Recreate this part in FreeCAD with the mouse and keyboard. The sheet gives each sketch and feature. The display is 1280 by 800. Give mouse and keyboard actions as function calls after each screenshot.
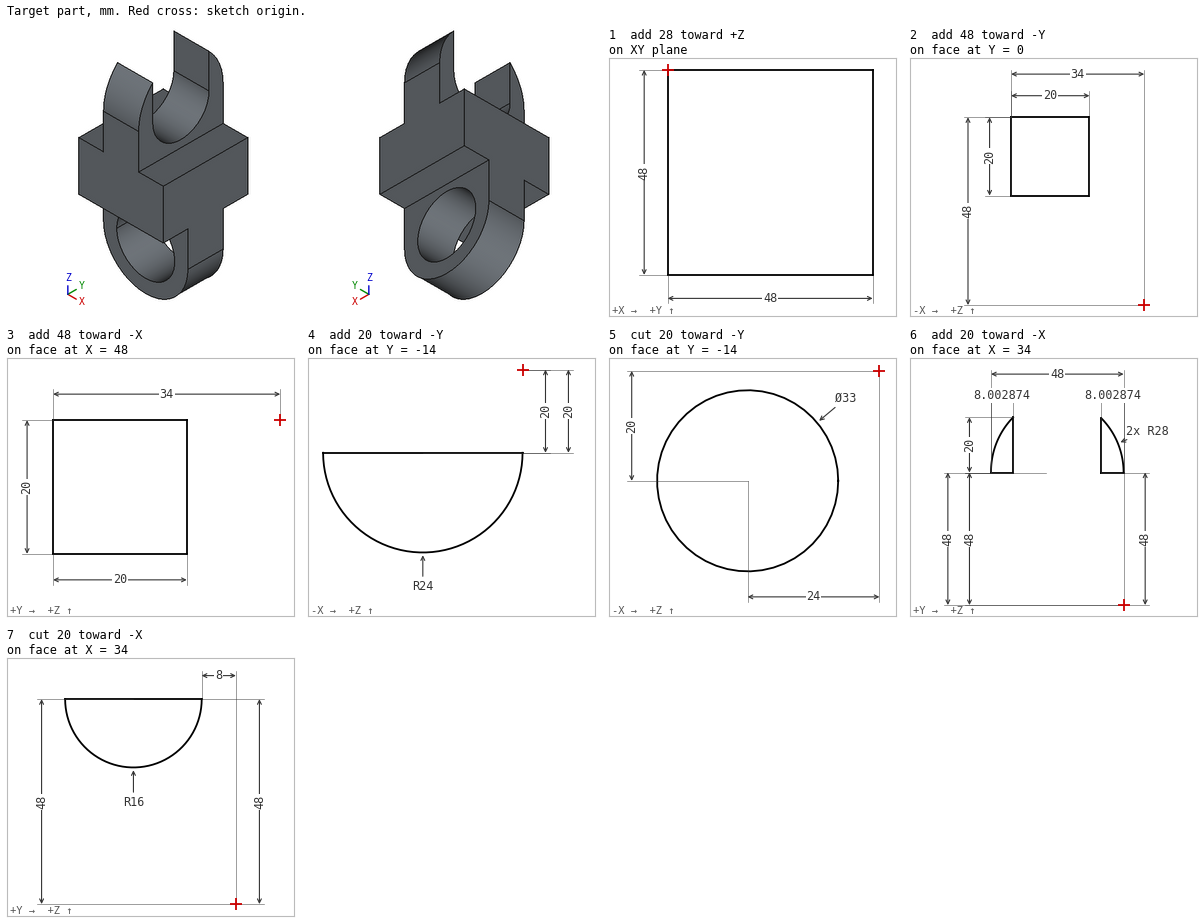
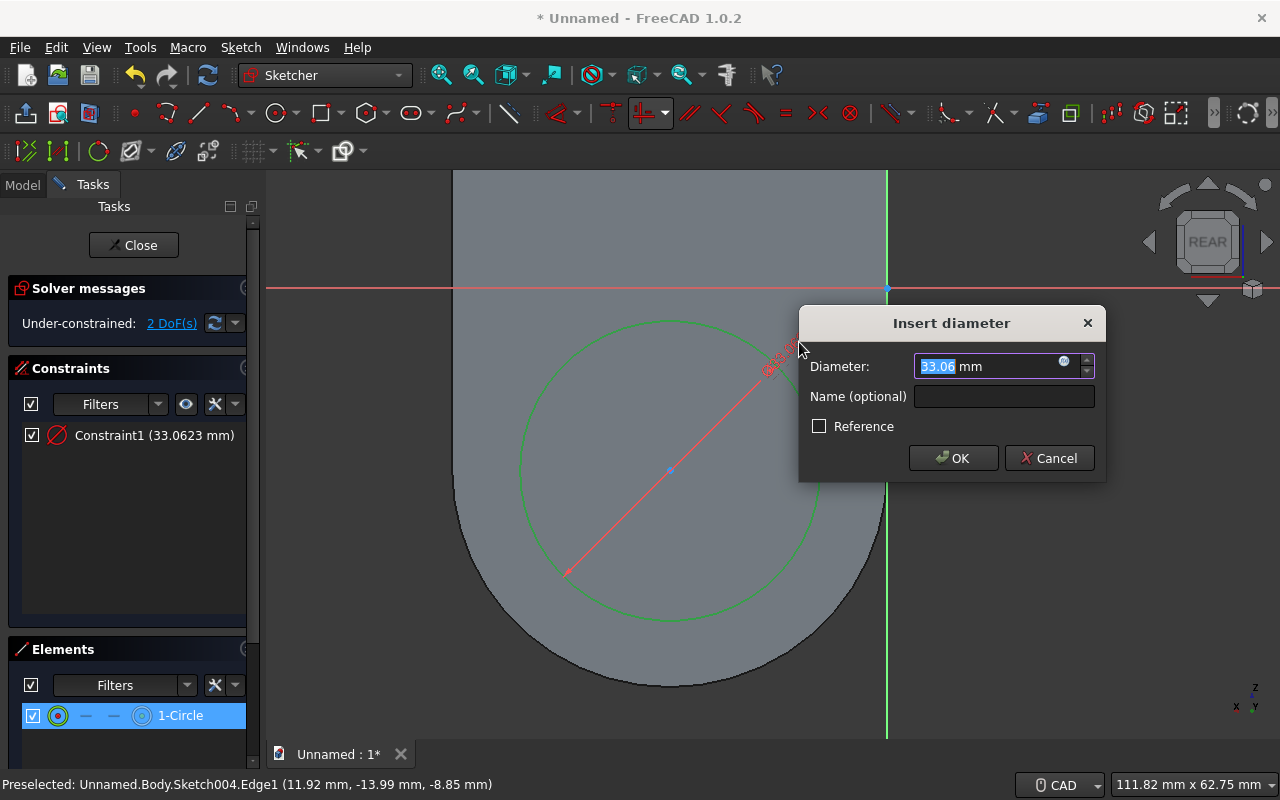
text(33)
key(Return)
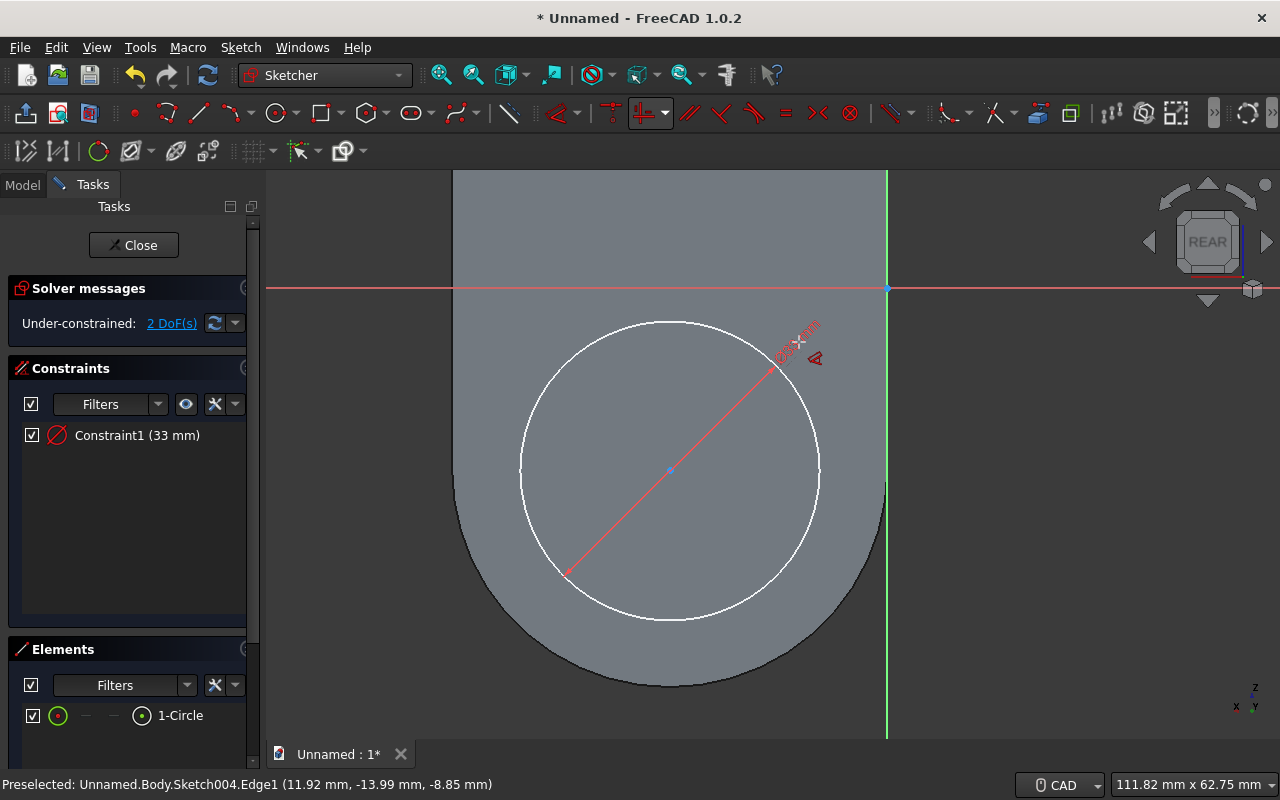
click(670, 471)
click(779, 254)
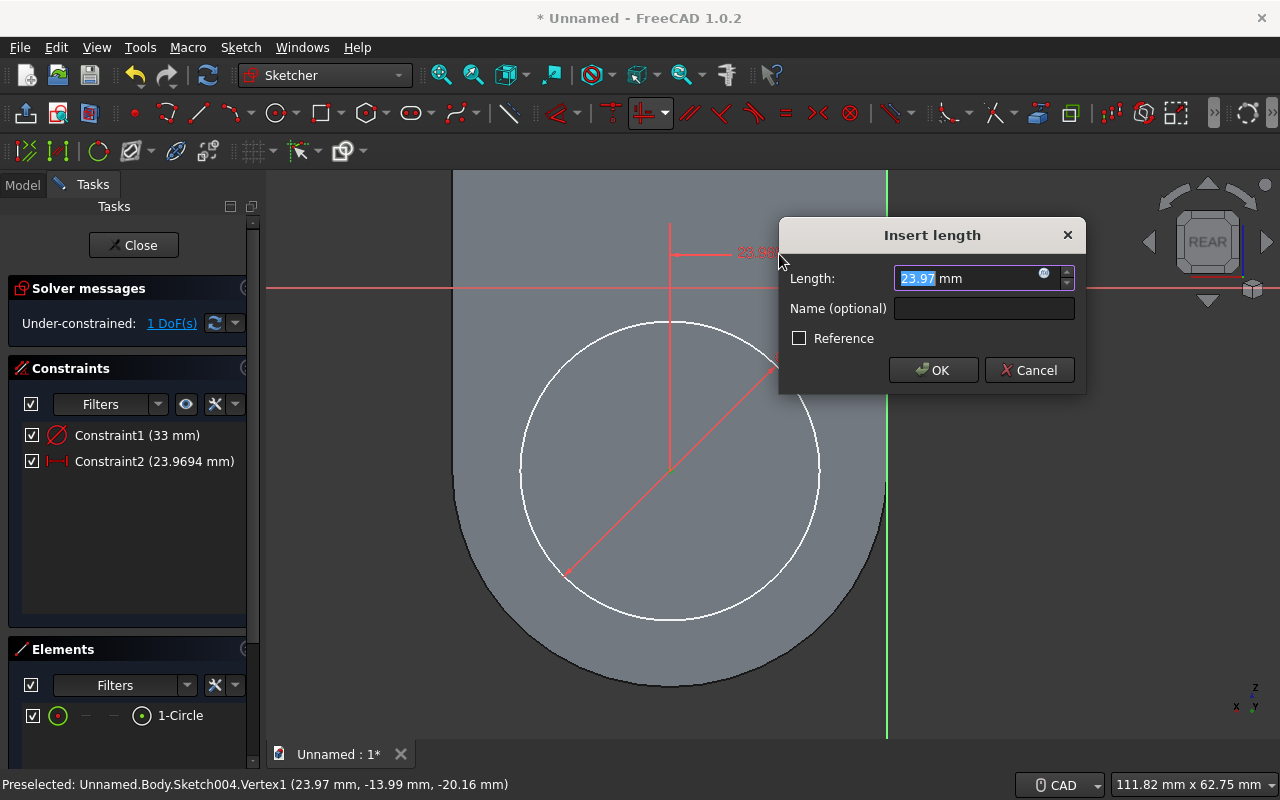
text(24)
key(Return)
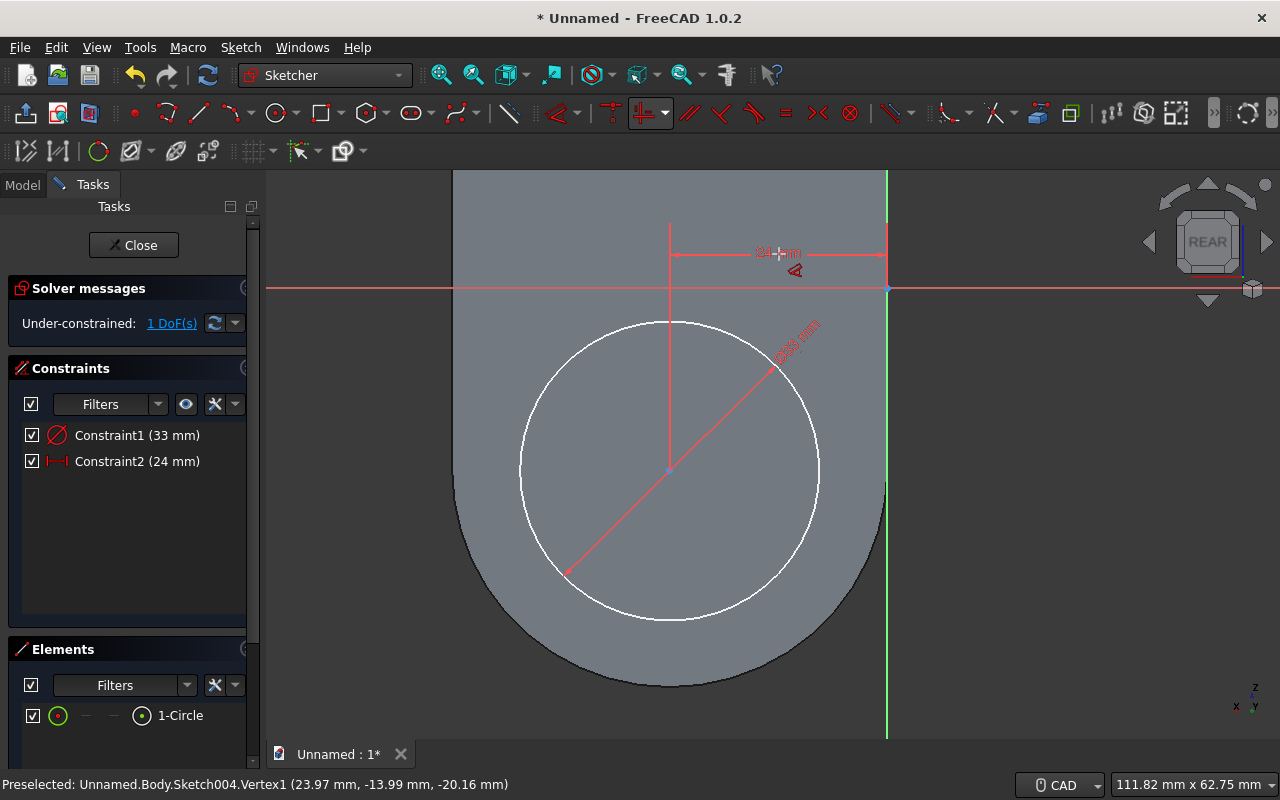
click(670, 471)
click(921, 380)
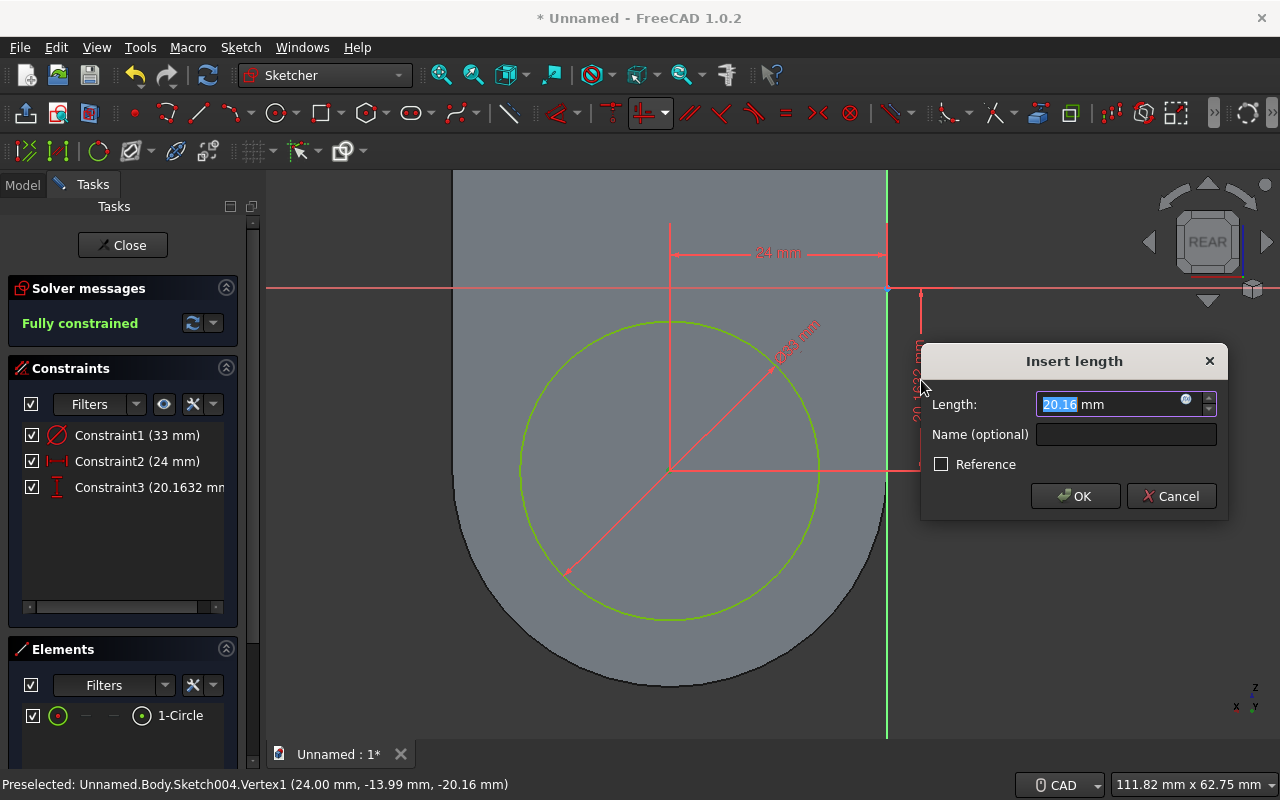
text(20)
key(Return)
key(Escape)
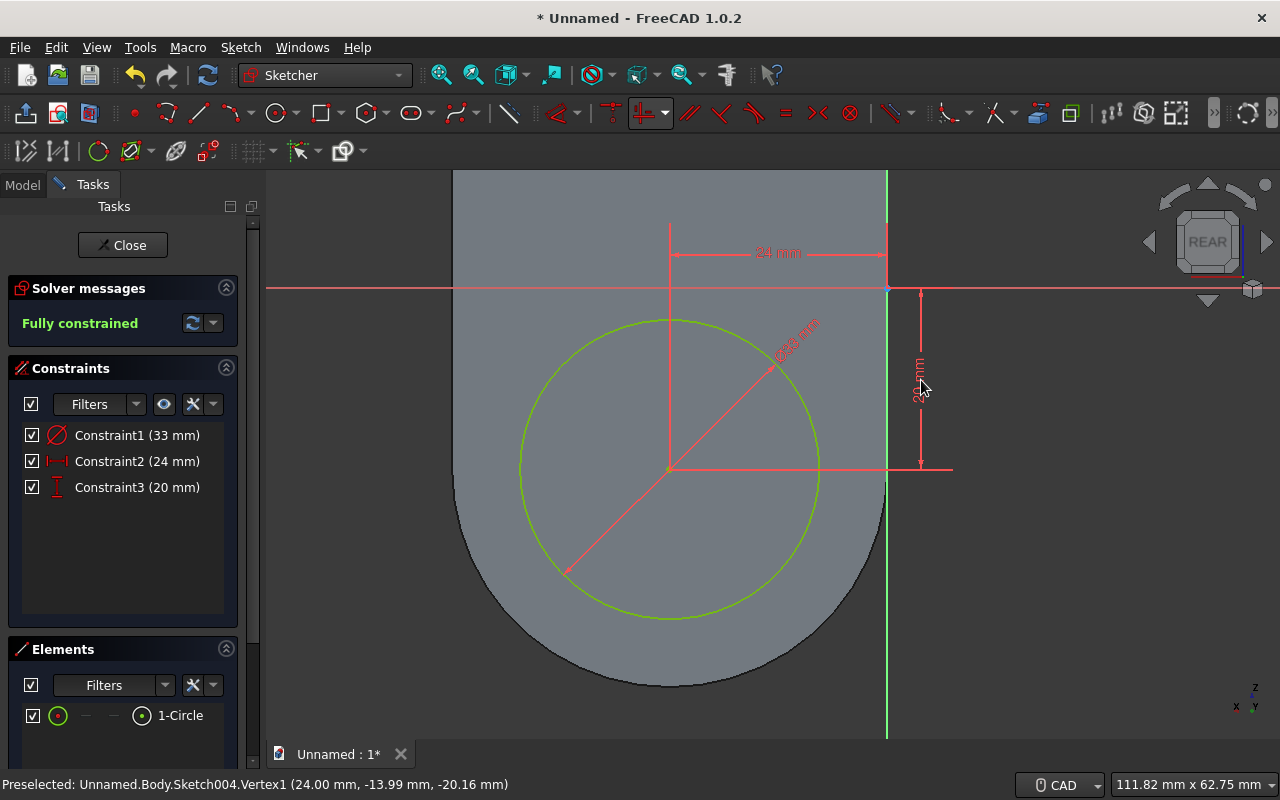
click(123, 245)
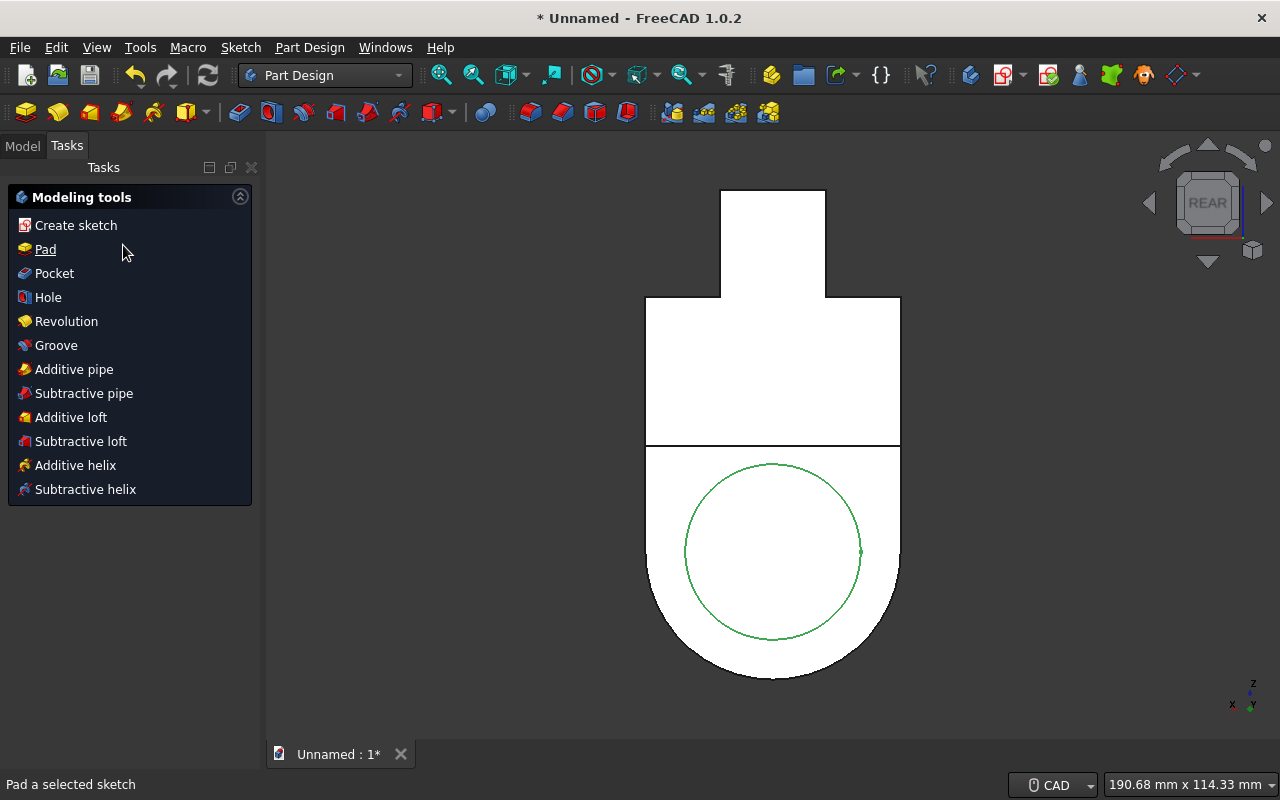
click(240, 112)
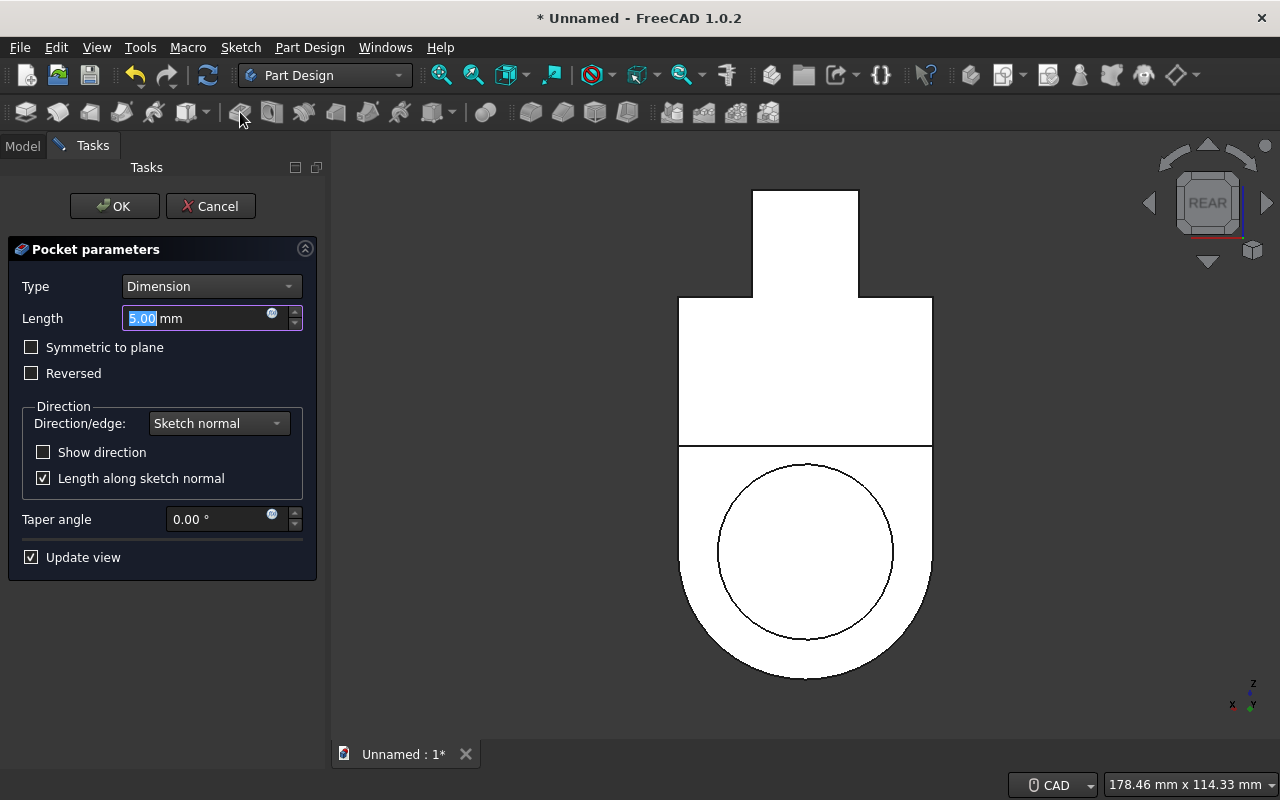
text(20)
key(Tab)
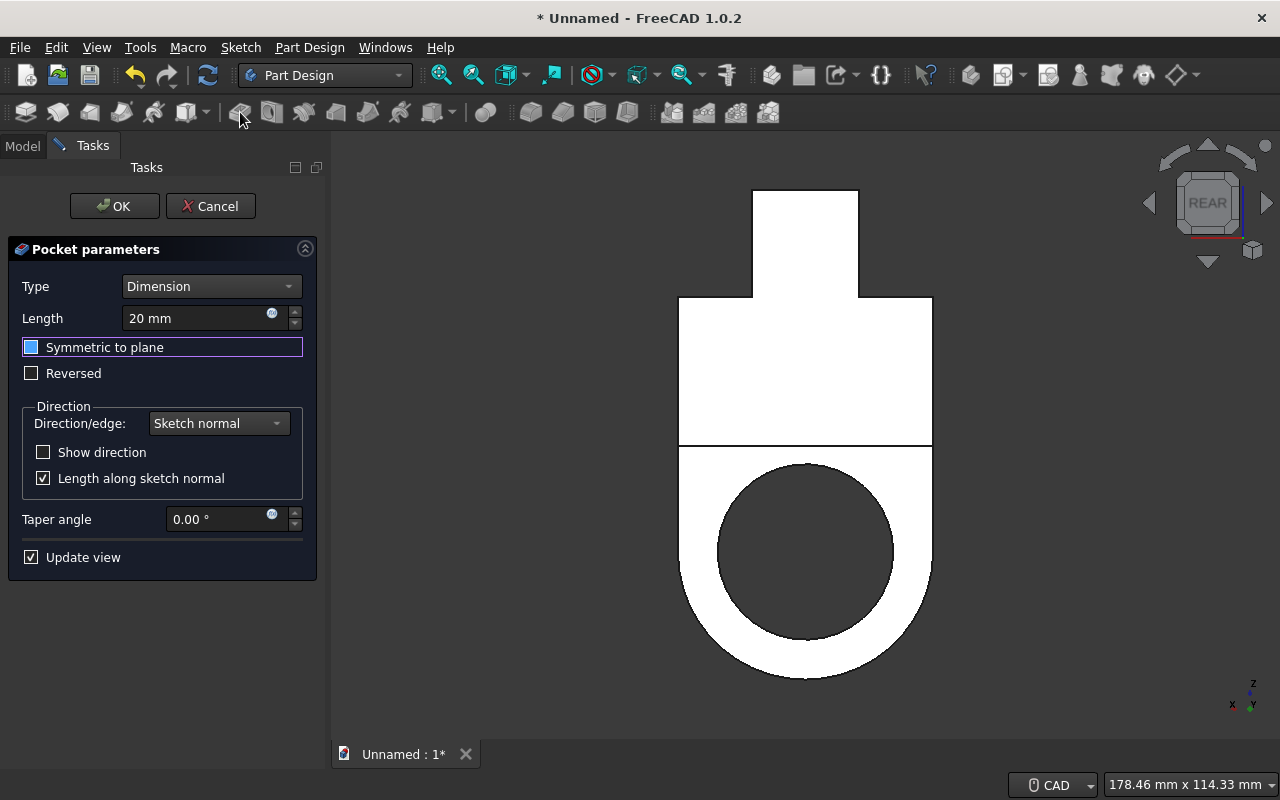
click(115, 206)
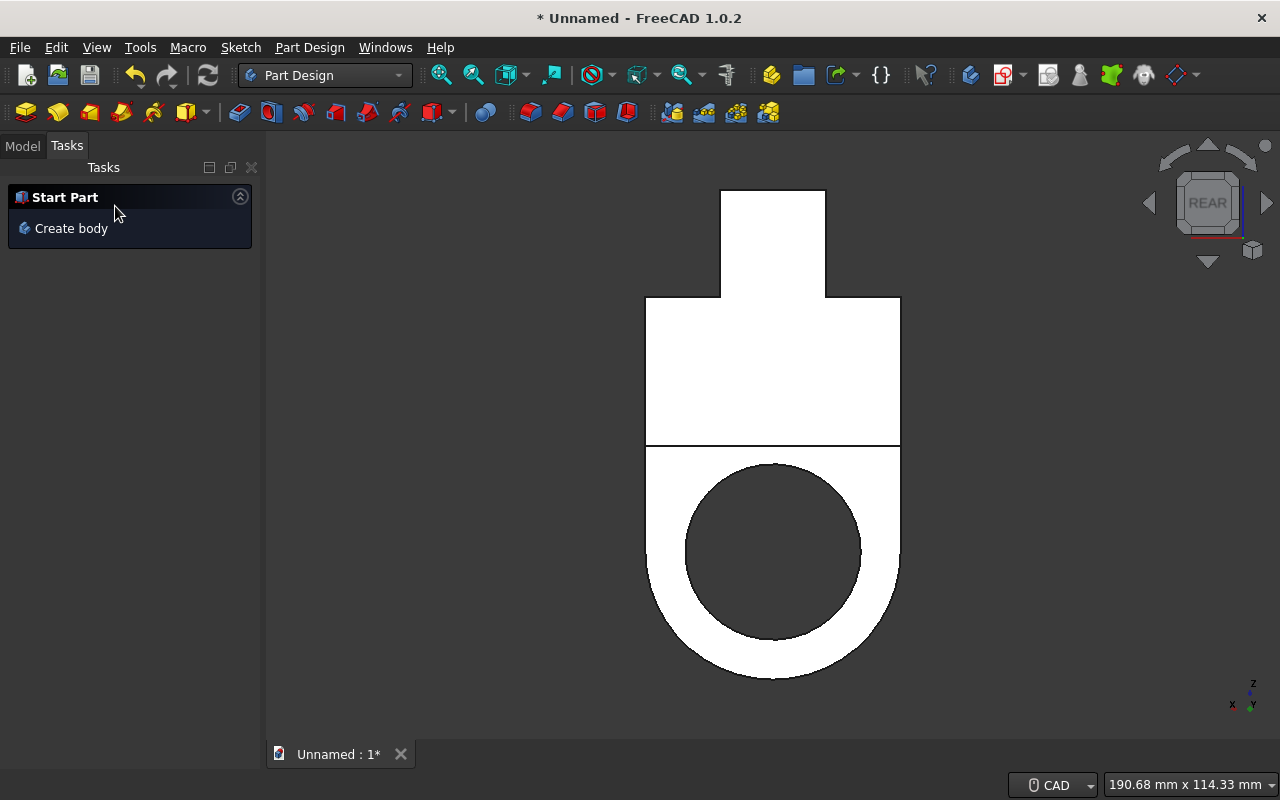
key(0)